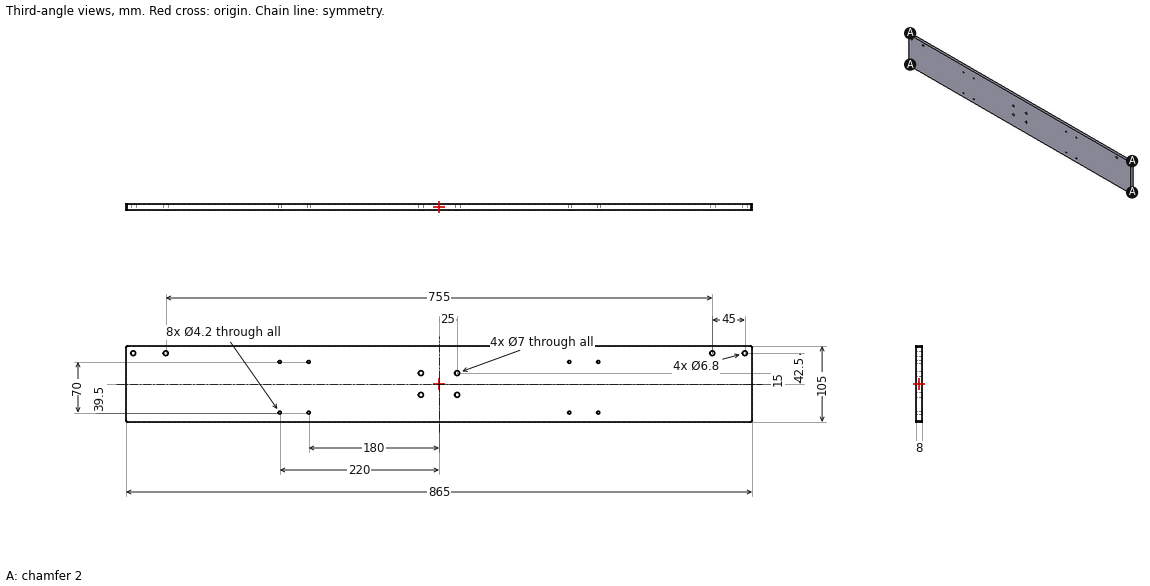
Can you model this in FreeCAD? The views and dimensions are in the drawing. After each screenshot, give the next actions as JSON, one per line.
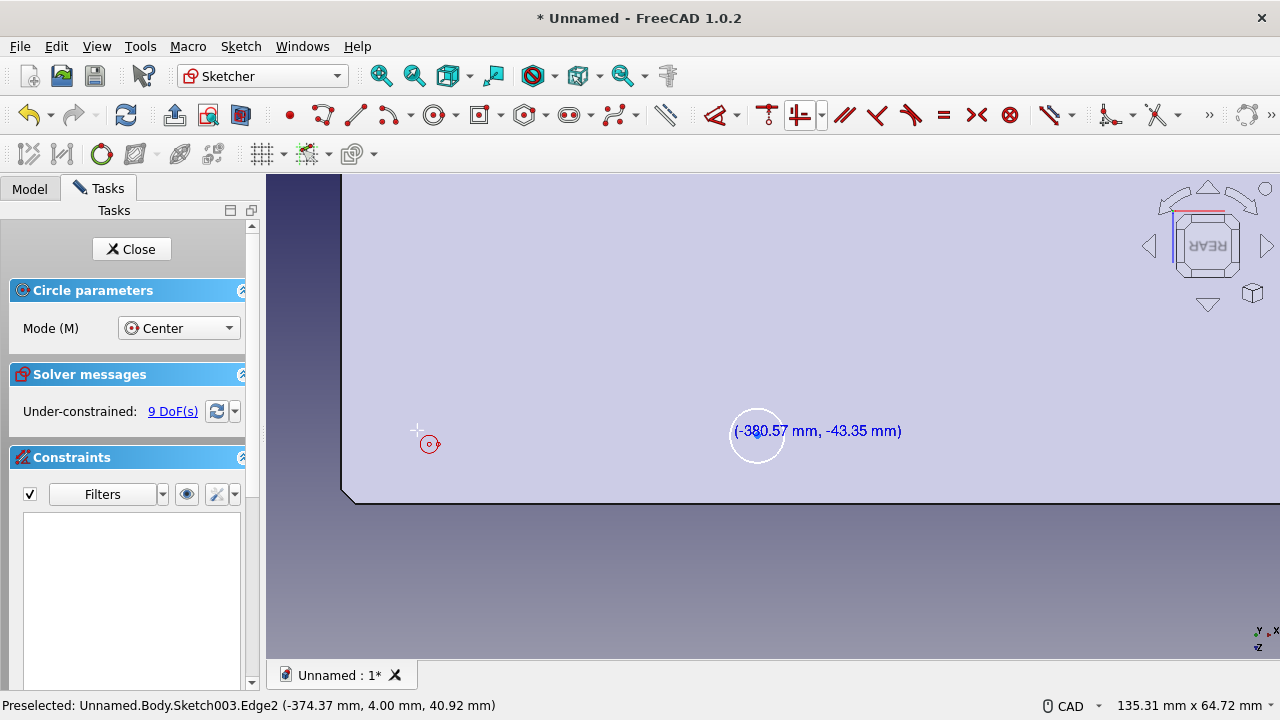
{"action": "scroll", "coordinate": [417, 430], "scroll_direction": "down", "scroll_amount": 12}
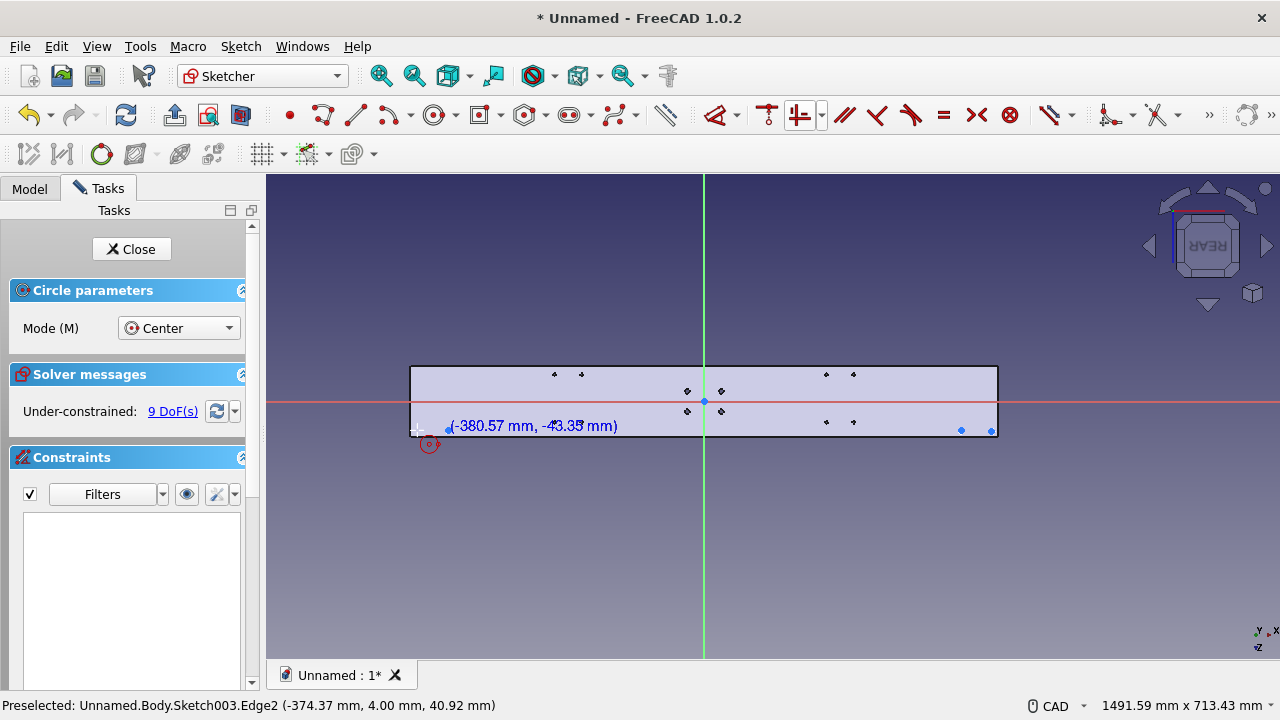
{"action": "left_click", "coordinate": [417, 430]}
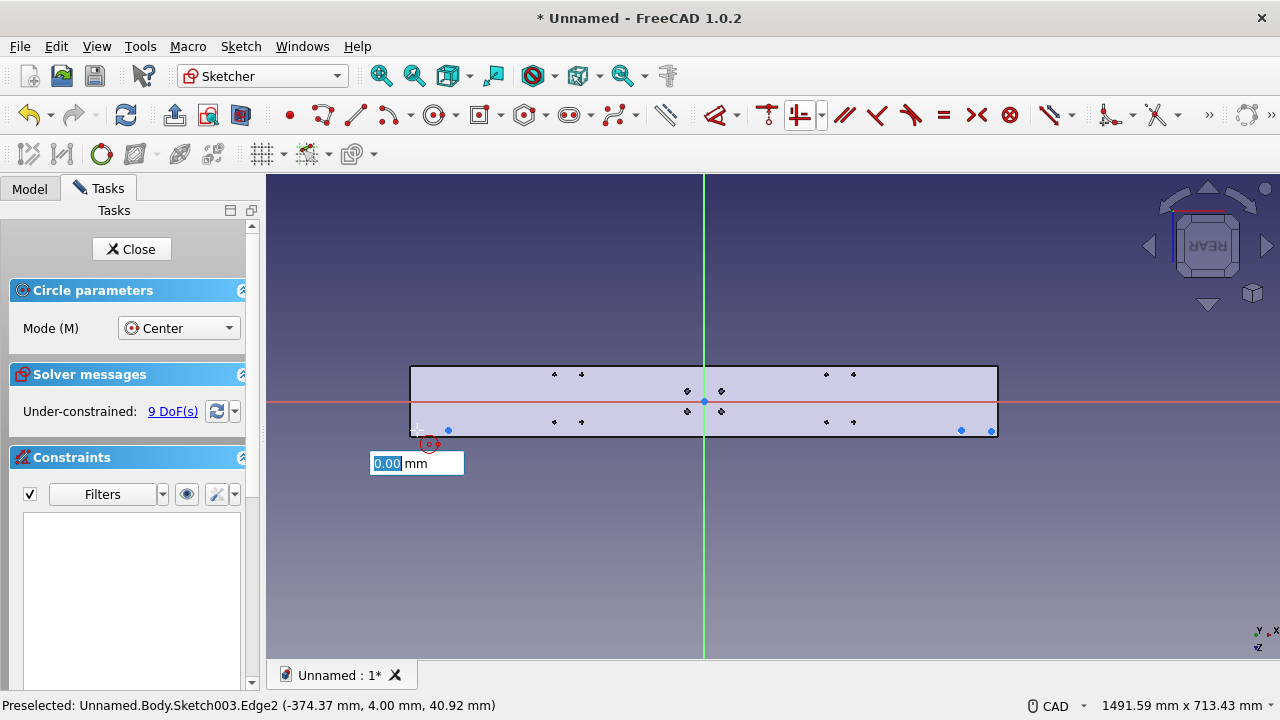
{"action": "scroll", "coordinate": [419, 429], "scroll_direction": "up", "scroll_amount": 10}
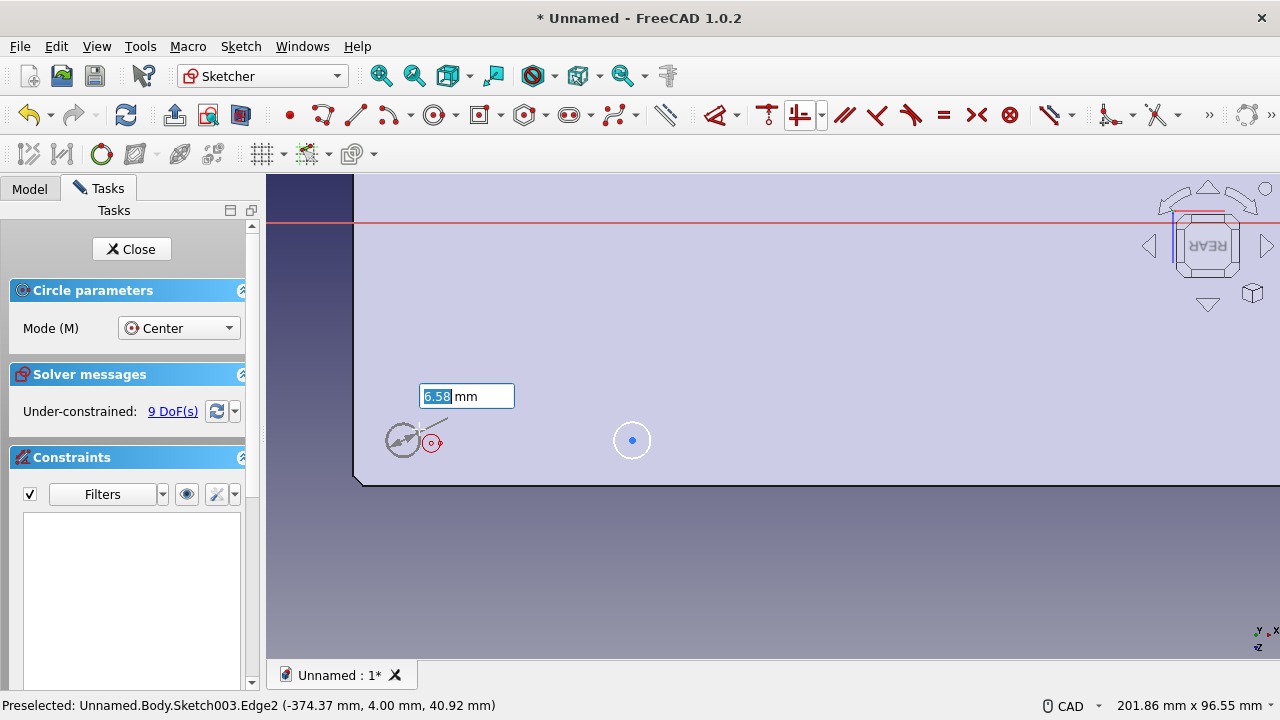
{"action": "left_click", "coordinate": [416, 424]}
{"action": "key", "text": "Escape"}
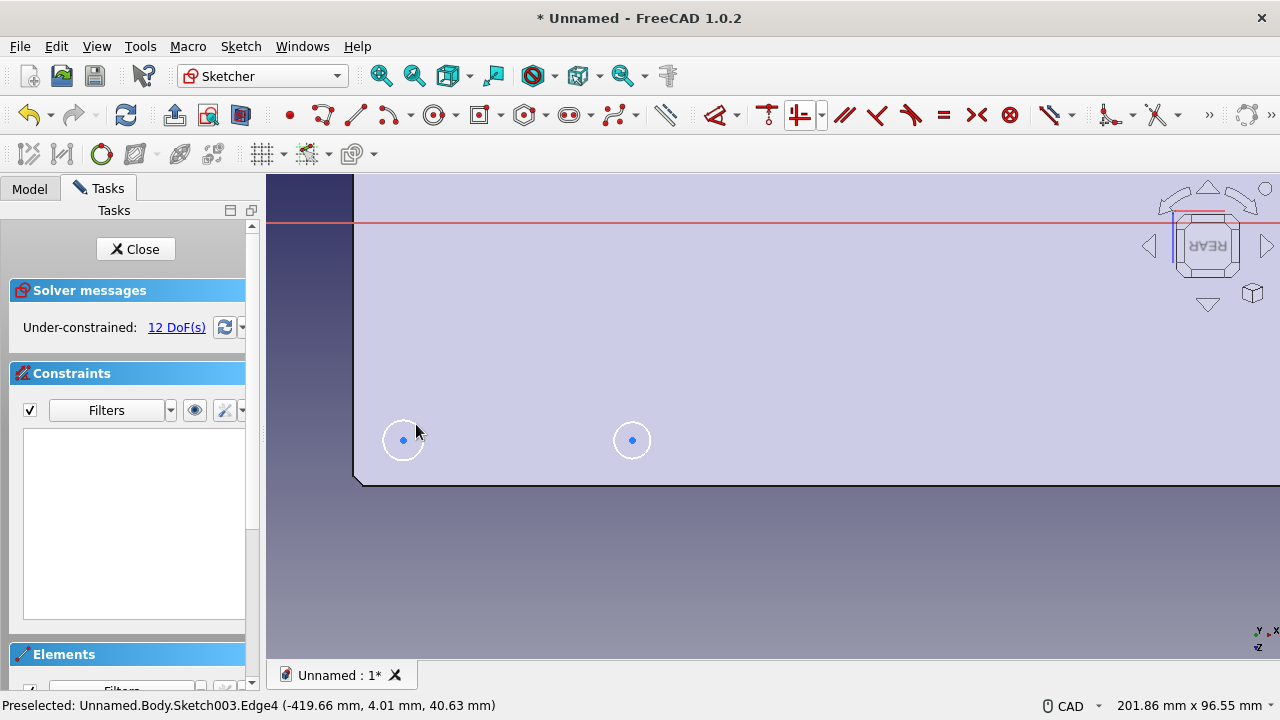
{"action": "scroll", "coordinate": [419, 429], "scroll_direction": "down", "scroll_amount": 10}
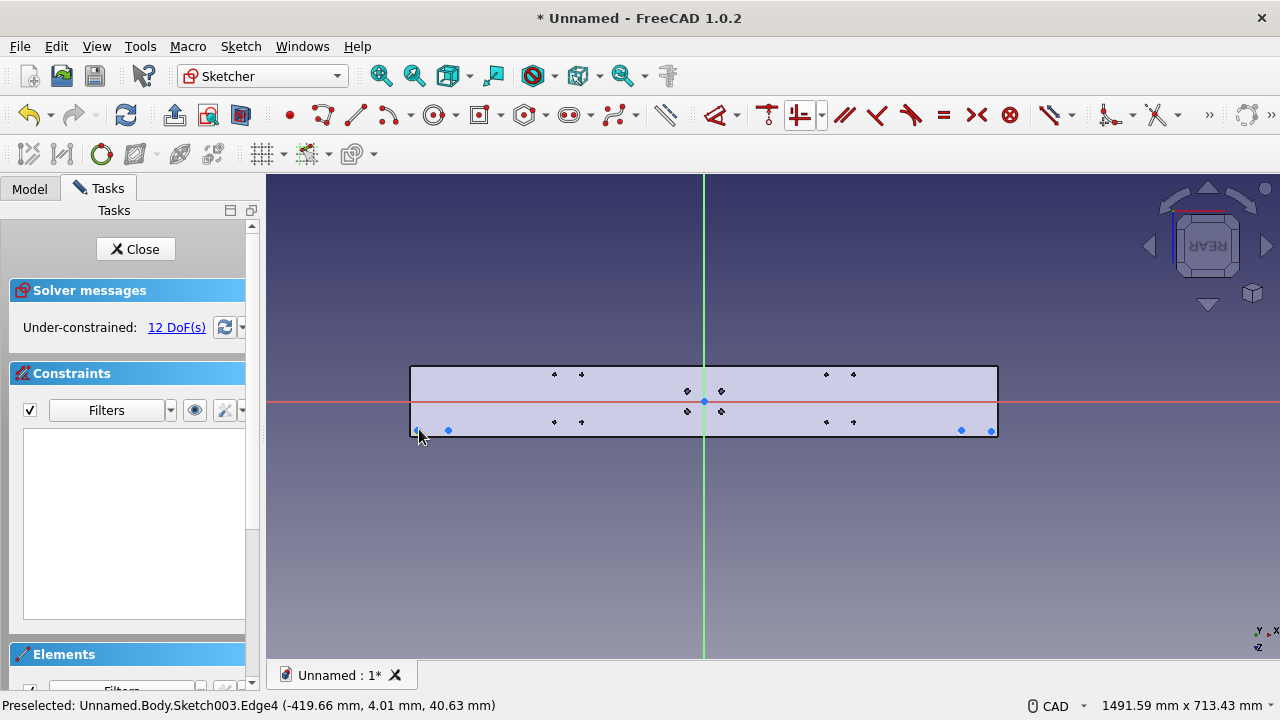
{"action": "scroll", "coordinate": [994, 429], "scroll_direction": "up", "scroll_amount": 9}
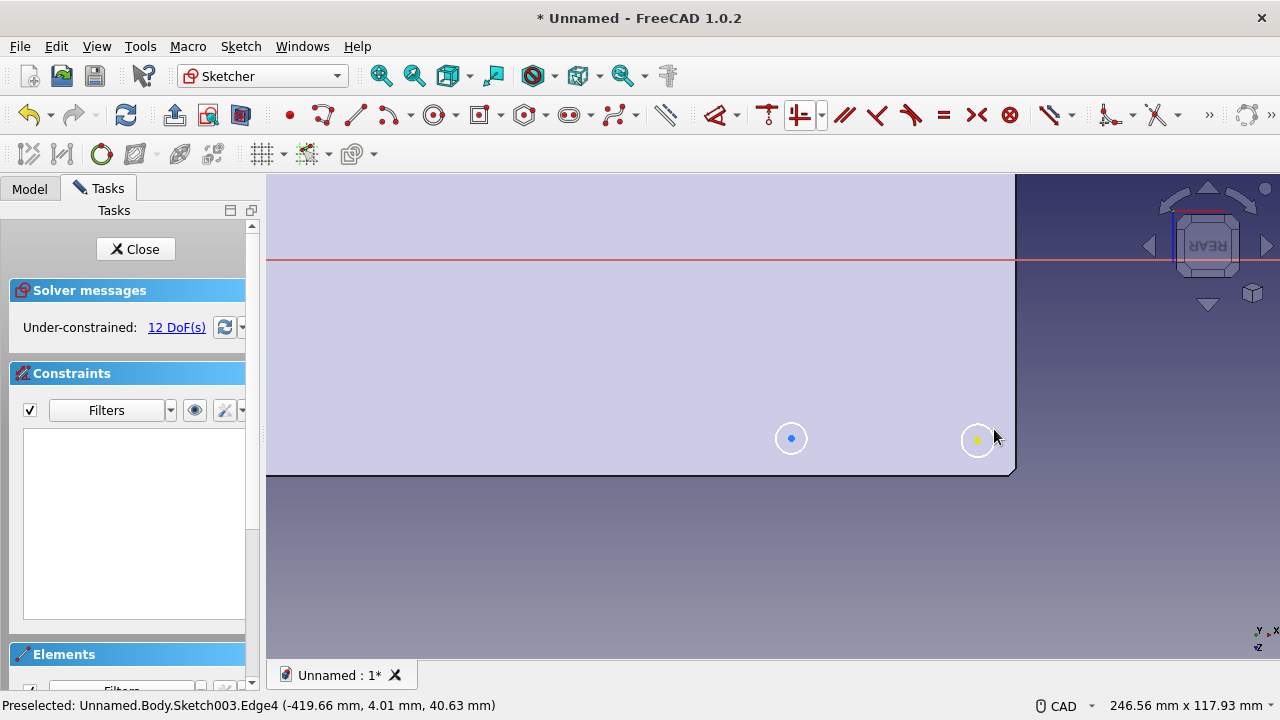
{"action": "left_click", "coordinate": [989, 429]}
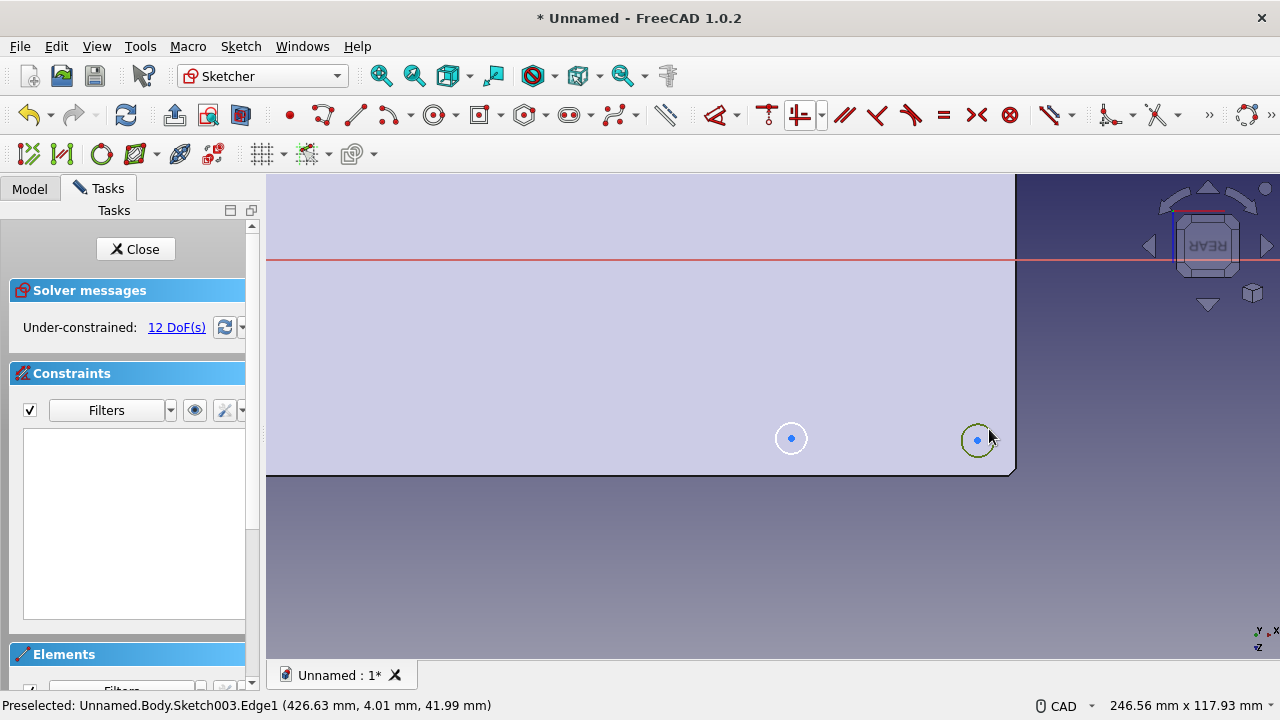
{"action": "left_click", "coordinate": [802, 428]}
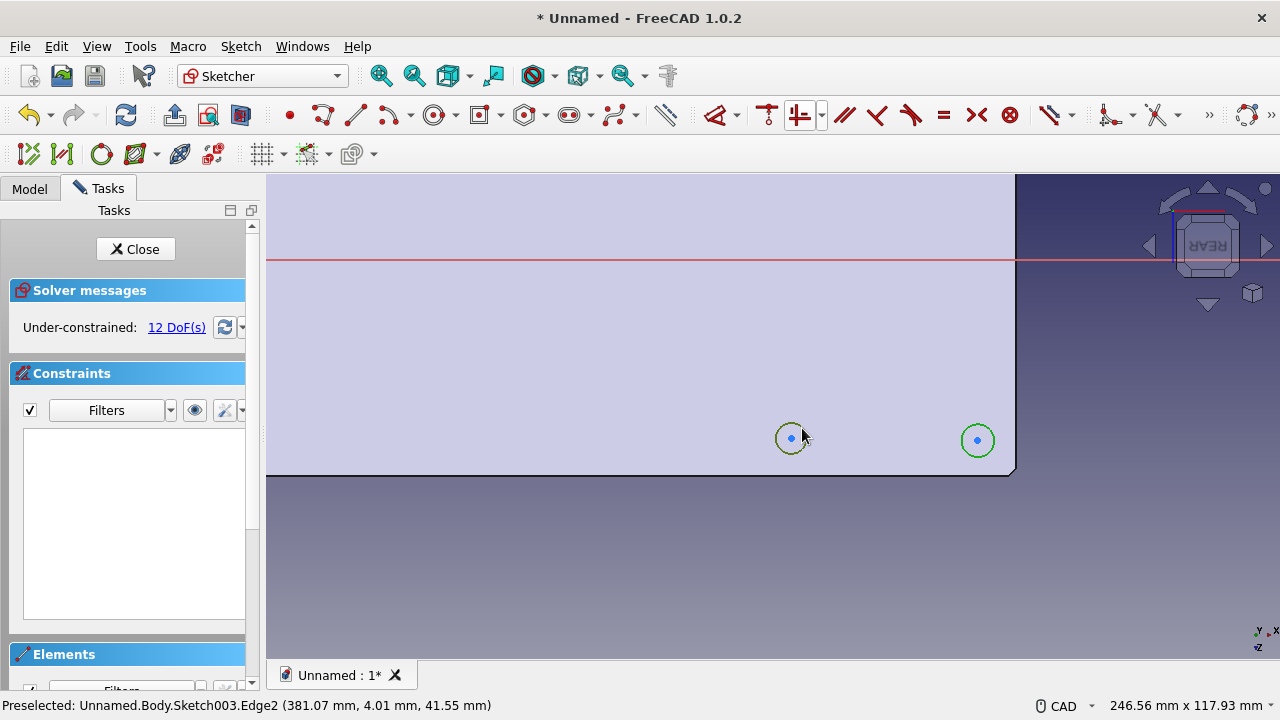
{"action": "scroll", "coordinate": [995, 429], "scroll_direction": "down", "scroll_amount": 9}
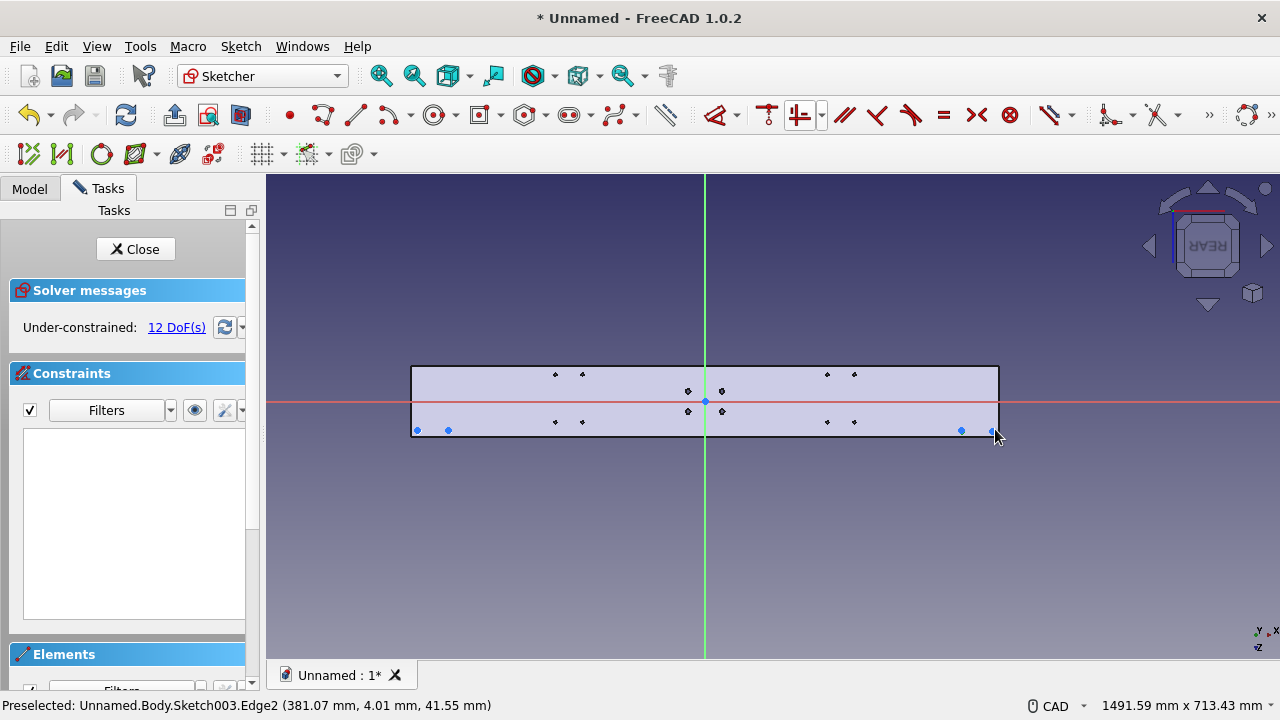
{"action": "scroll", "coordinate": [451, 429], "scroll_direction": "up", "scroll_amount": 9}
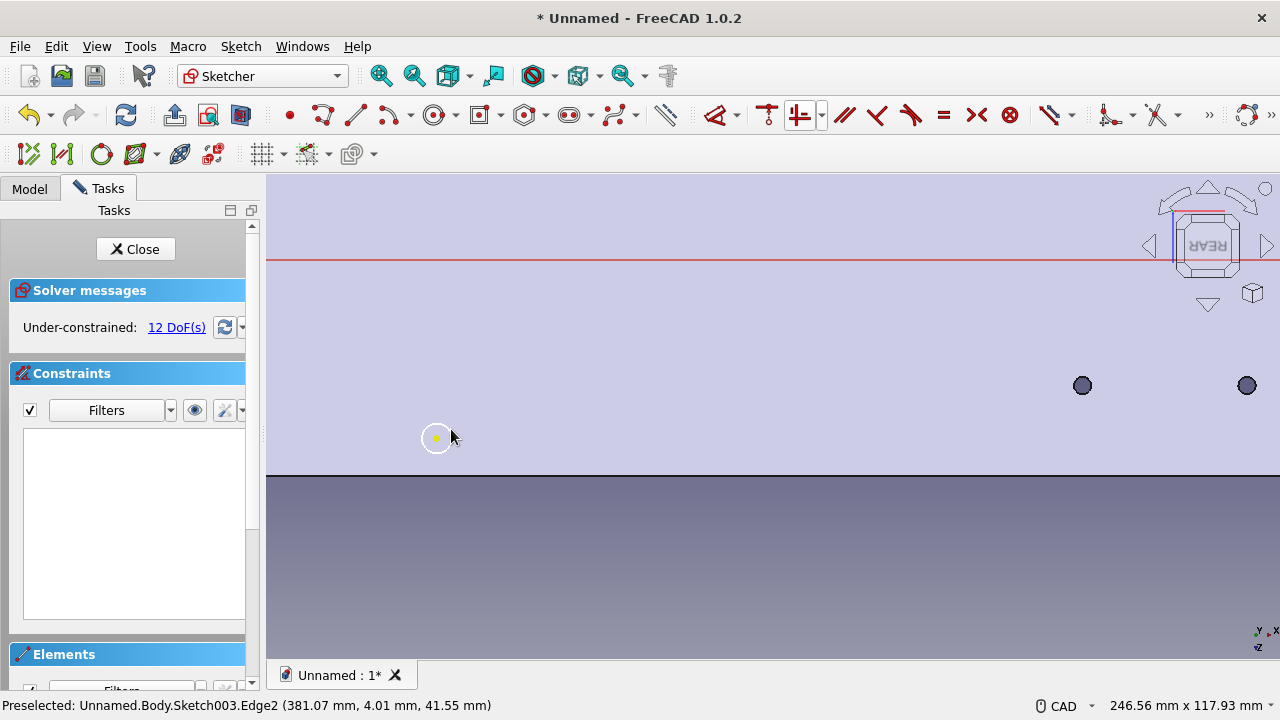
{"action": "left_click", "coordinate": [447, 428]}